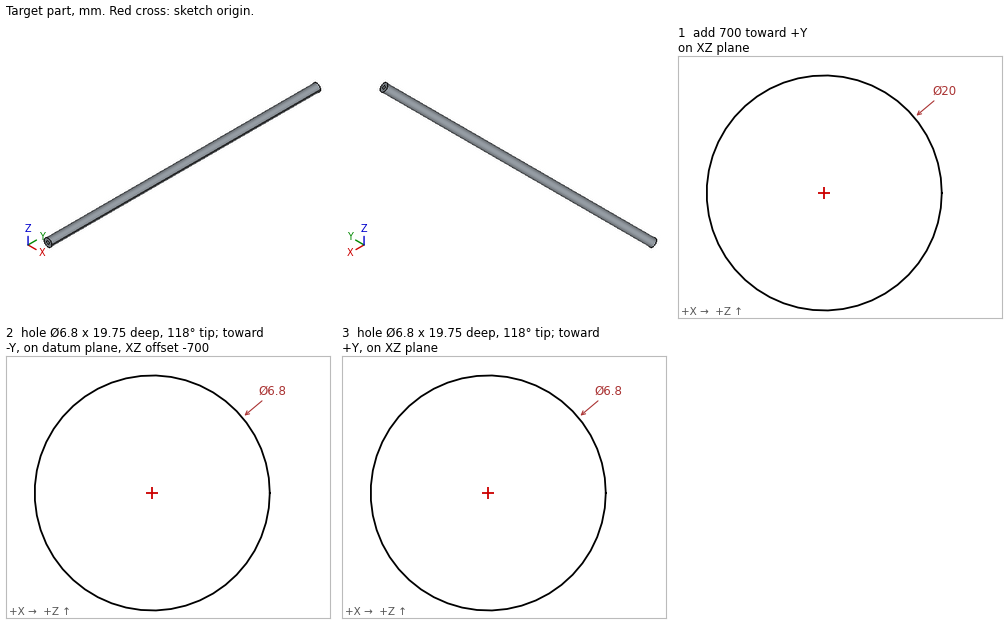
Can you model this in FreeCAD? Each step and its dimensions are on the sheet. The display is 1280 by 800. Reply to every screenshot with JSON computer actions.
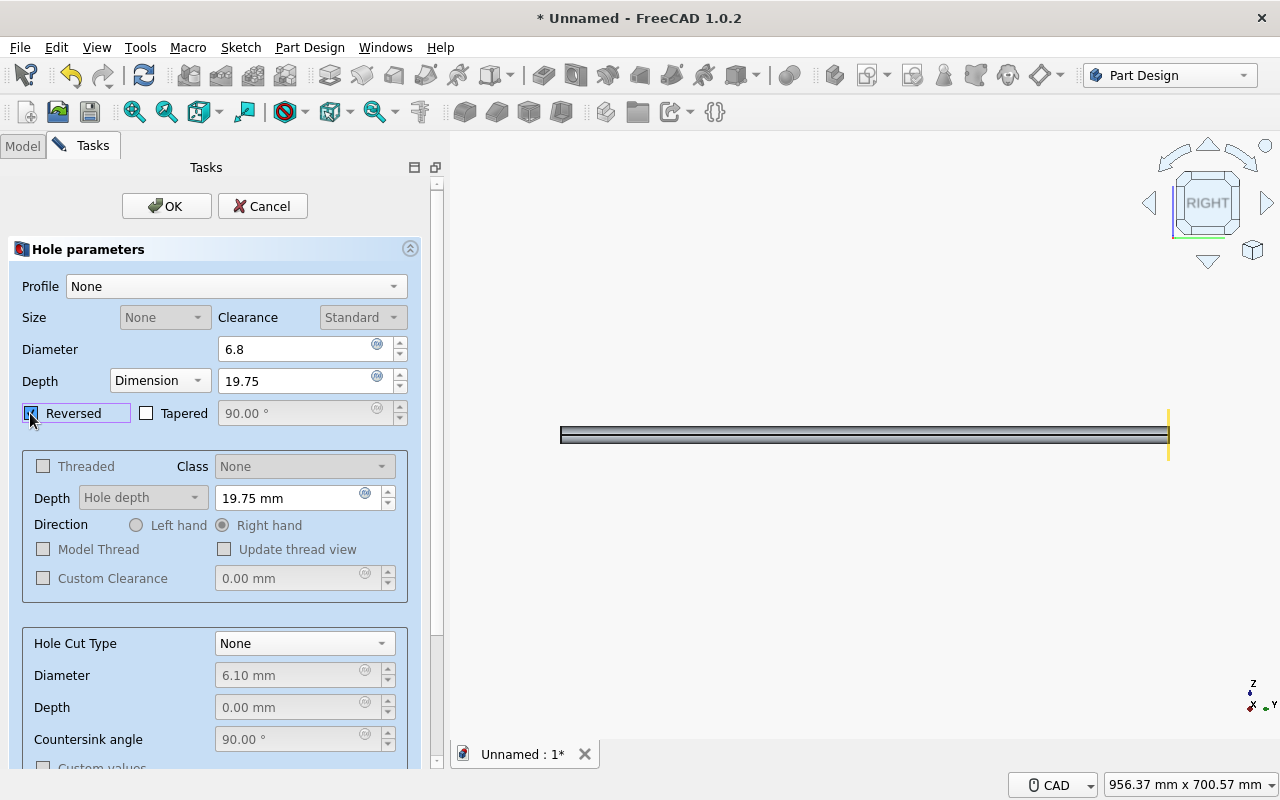
{"action": "left_click", "coordinate": [167, 206]}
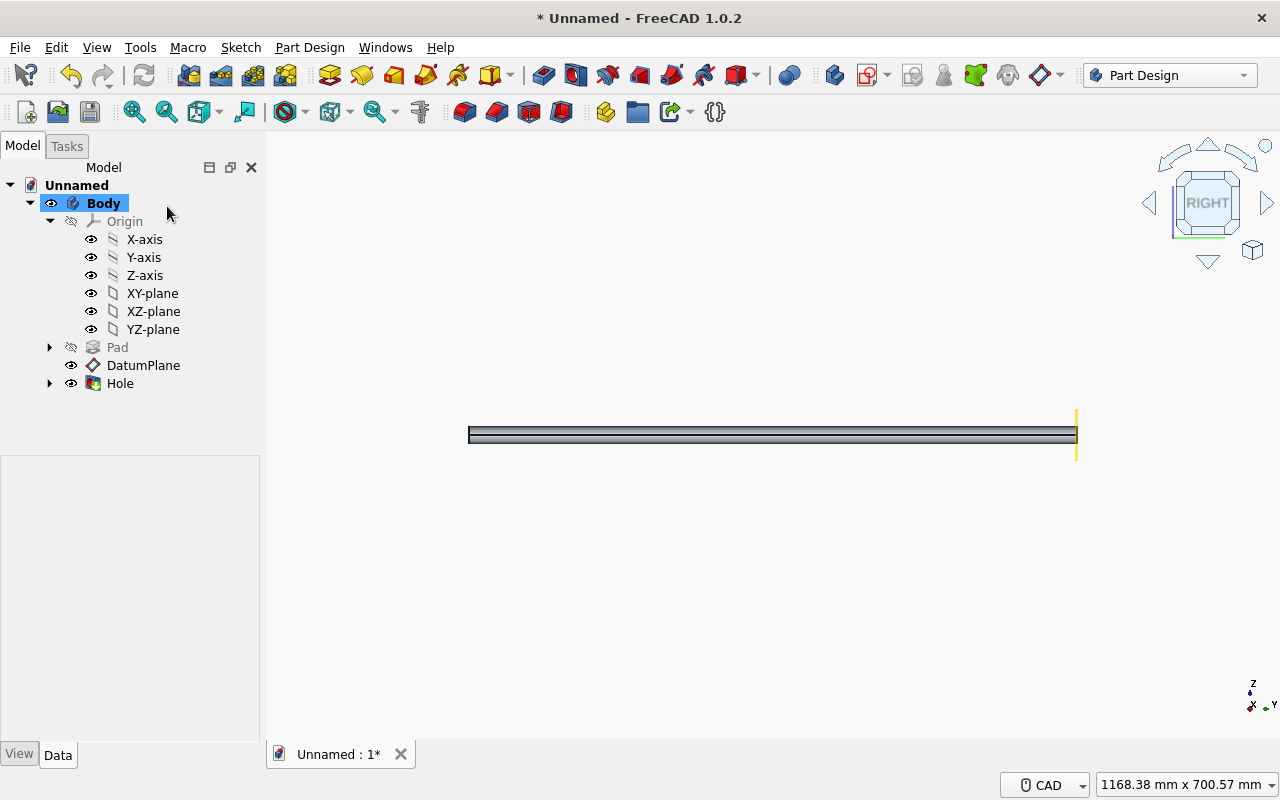
{"action": "left_click", "coordinate": [116, 365]}
{"action": "key", "text": "space"}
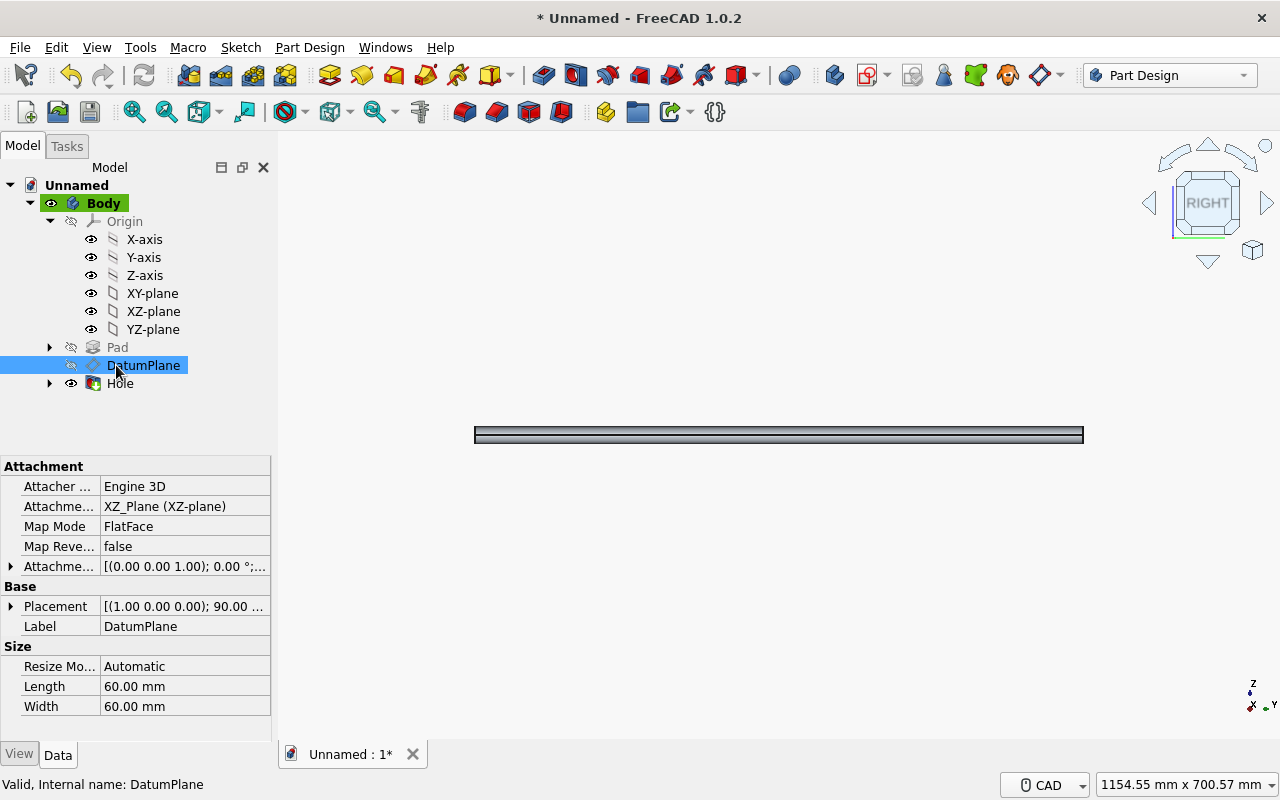
{"action": "left_click", "coordinate": [318, 699]}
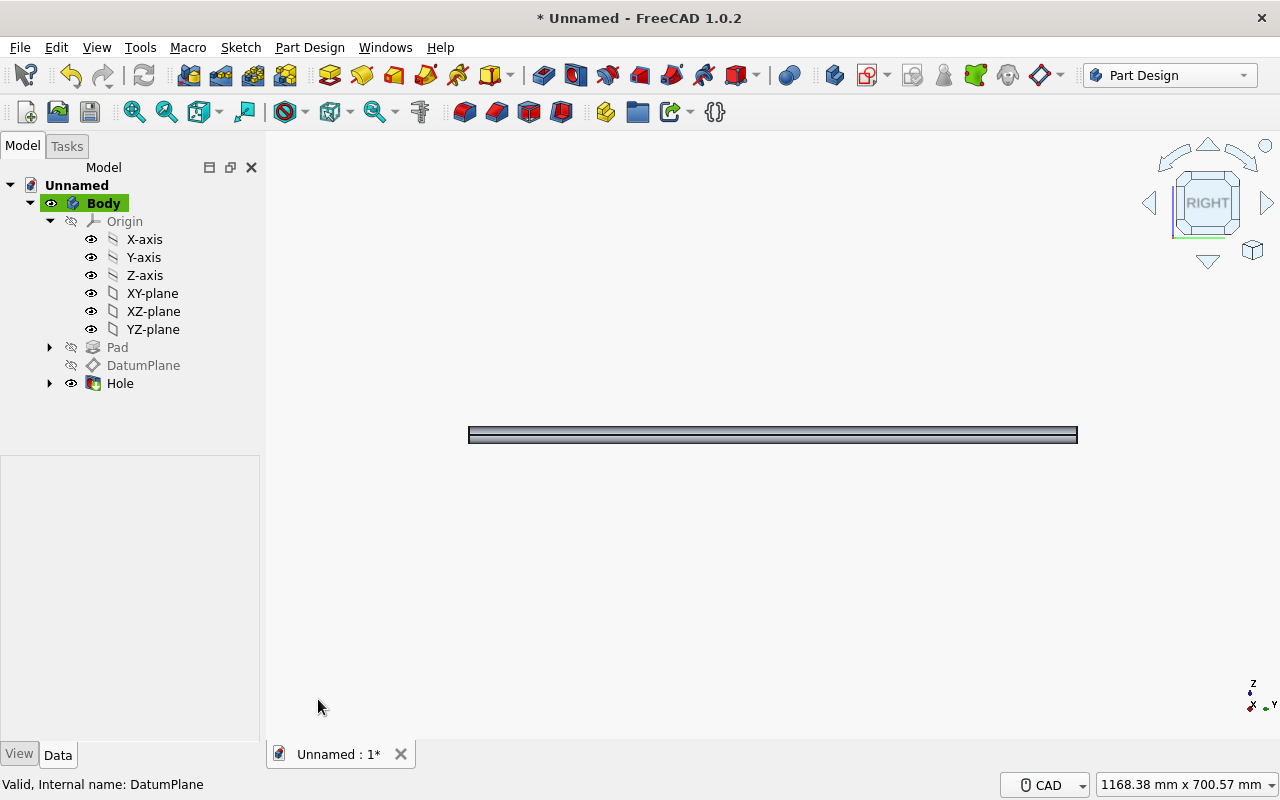
{"action": "left_click", "coordinate": [868, 76]}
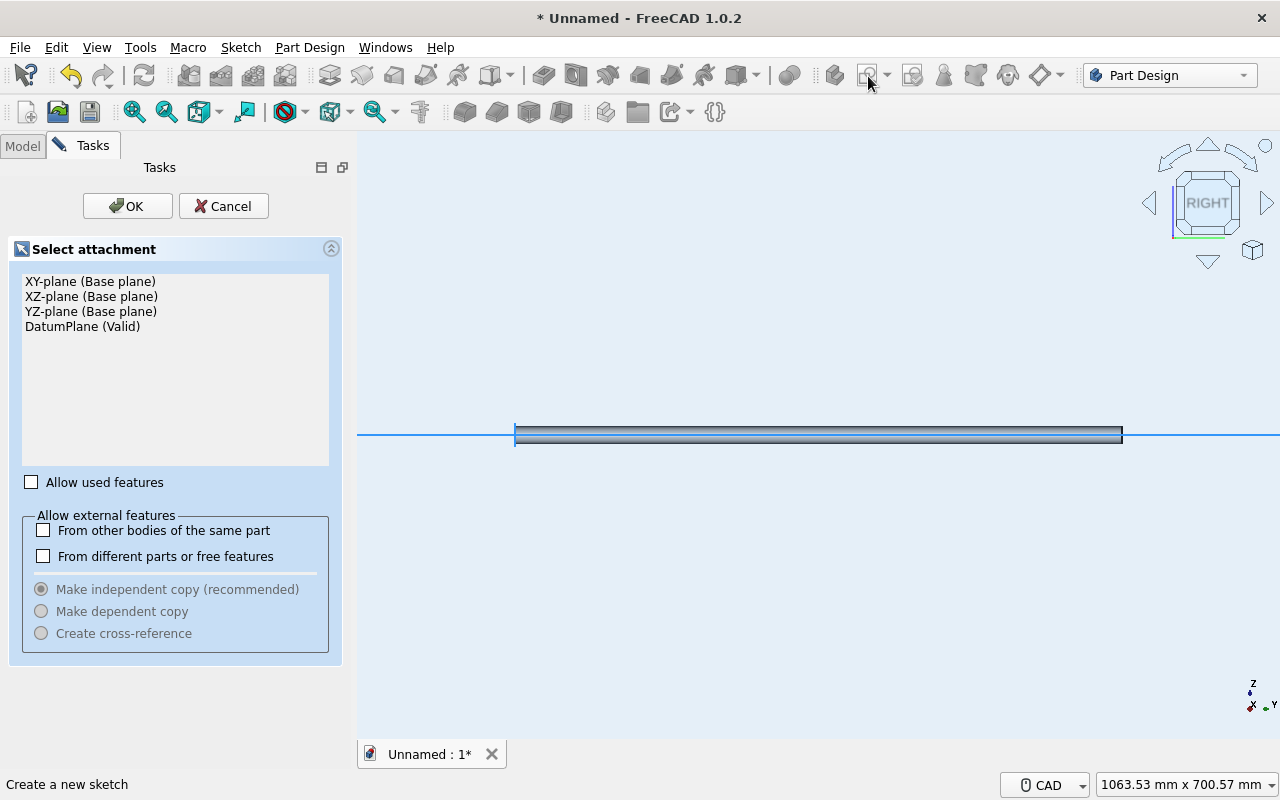
{"action": "left_click", "coordinate": [82, 296]}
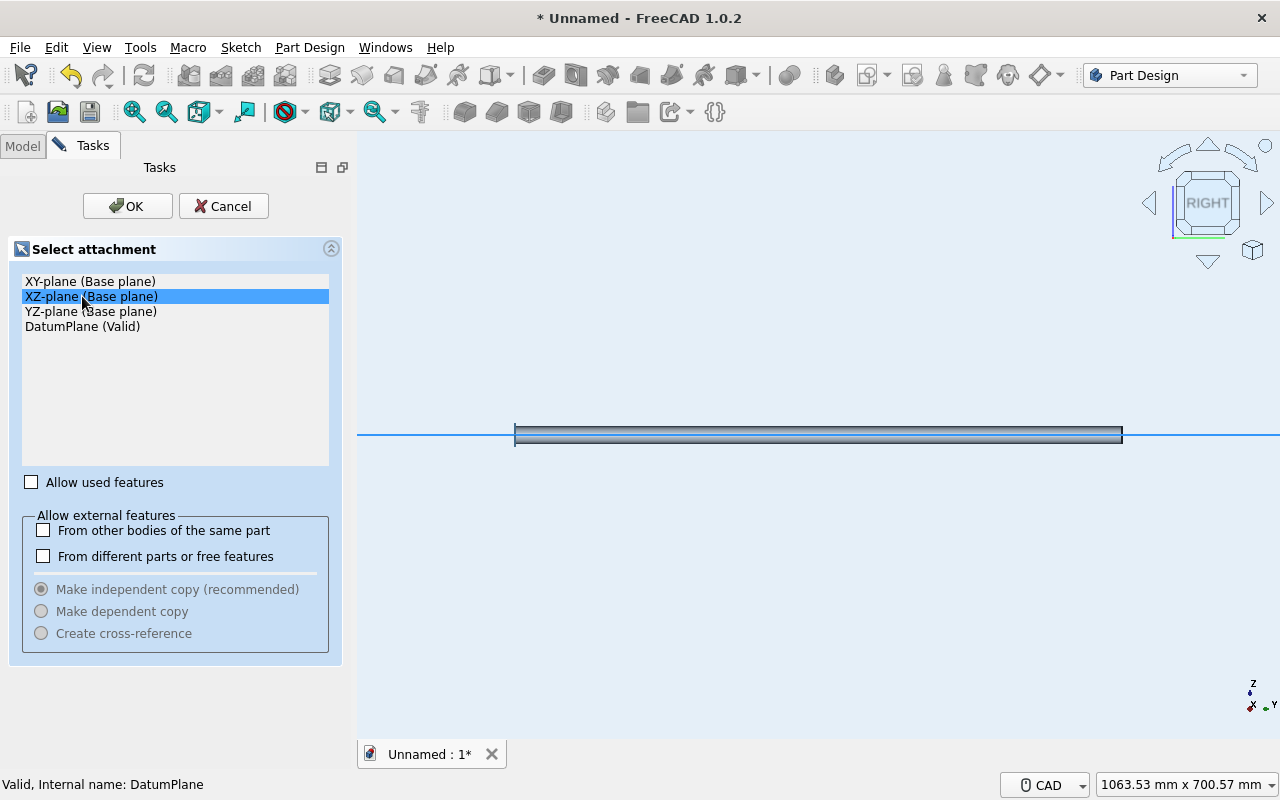
{"action": "left_click", "coordinate": [128, 206]}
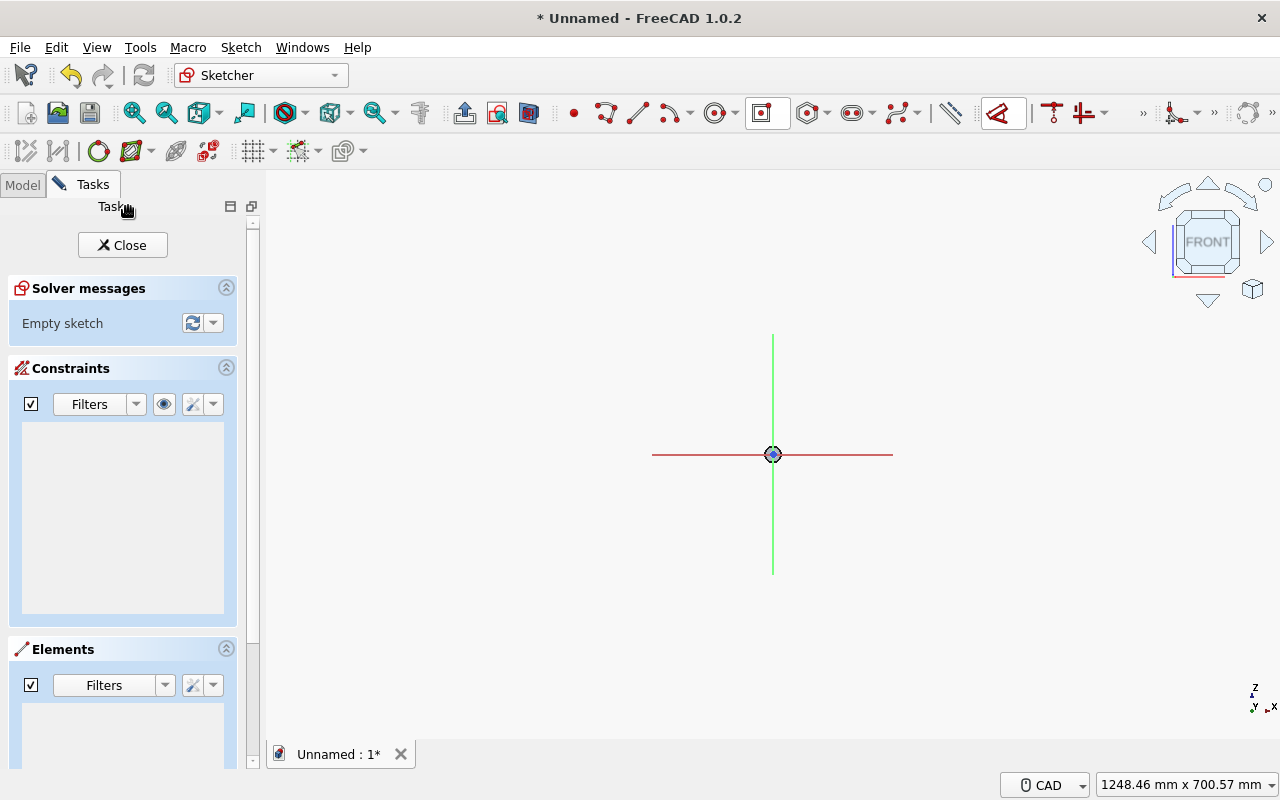
{"action": "scroll", "coordinate": [777, 455], "scroll_direction": "up", "scroll_amount": 15}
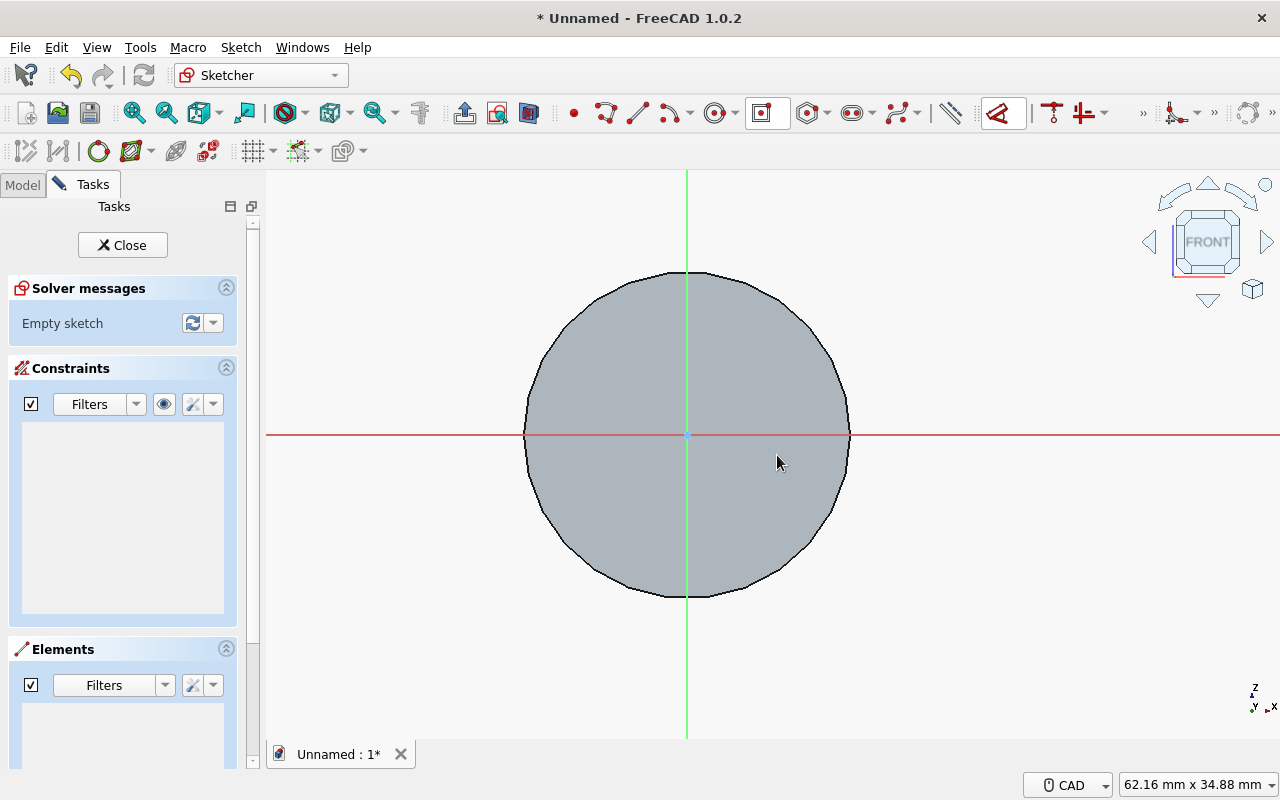
{"action": "scroll", "coordinate": [680, 427], "scroll_direction": "up", "scroll_amount": 6}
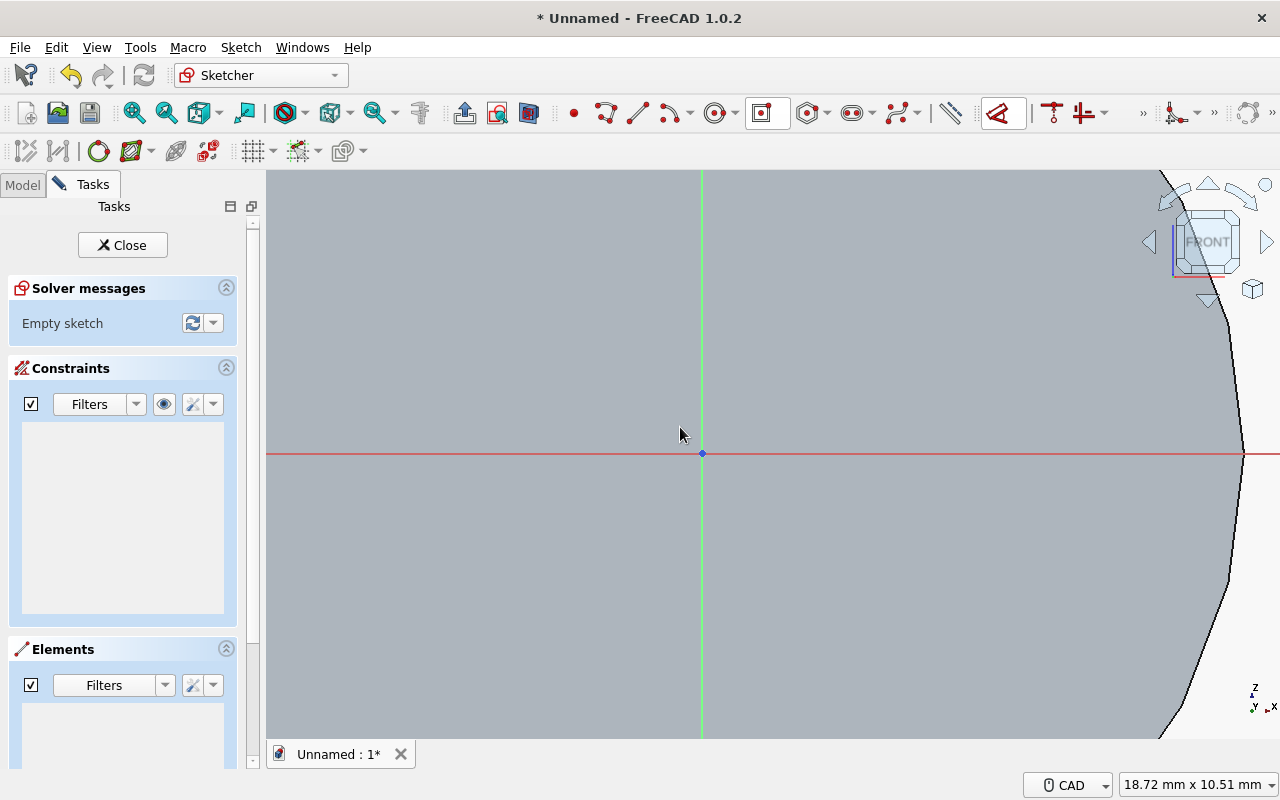
{"action": "left_click", "coordinate": [716, 114]}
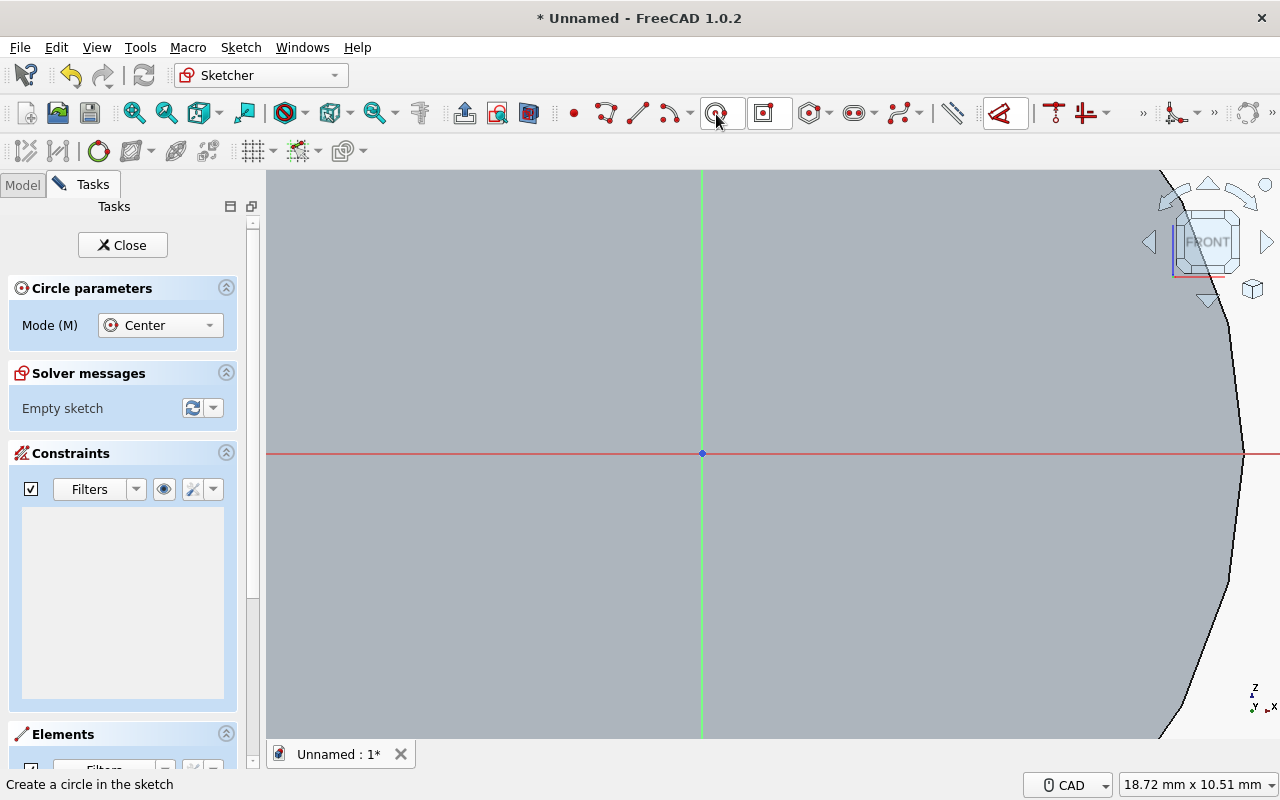
{"action": "left_click", "coordinate": [702, 454]}
{"action": "mouse_move", "coordinate": [833, 324]}